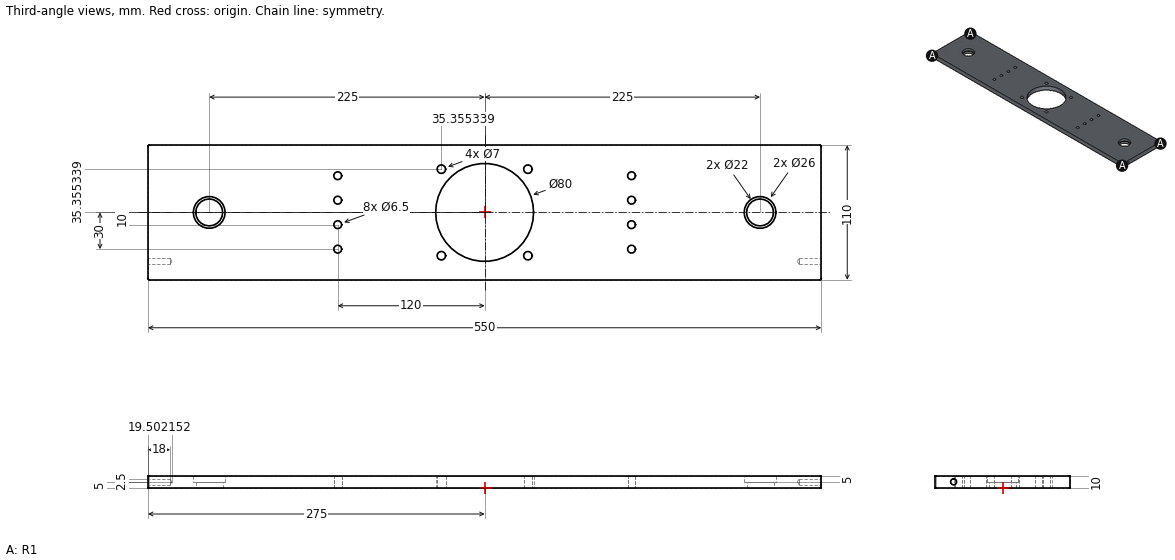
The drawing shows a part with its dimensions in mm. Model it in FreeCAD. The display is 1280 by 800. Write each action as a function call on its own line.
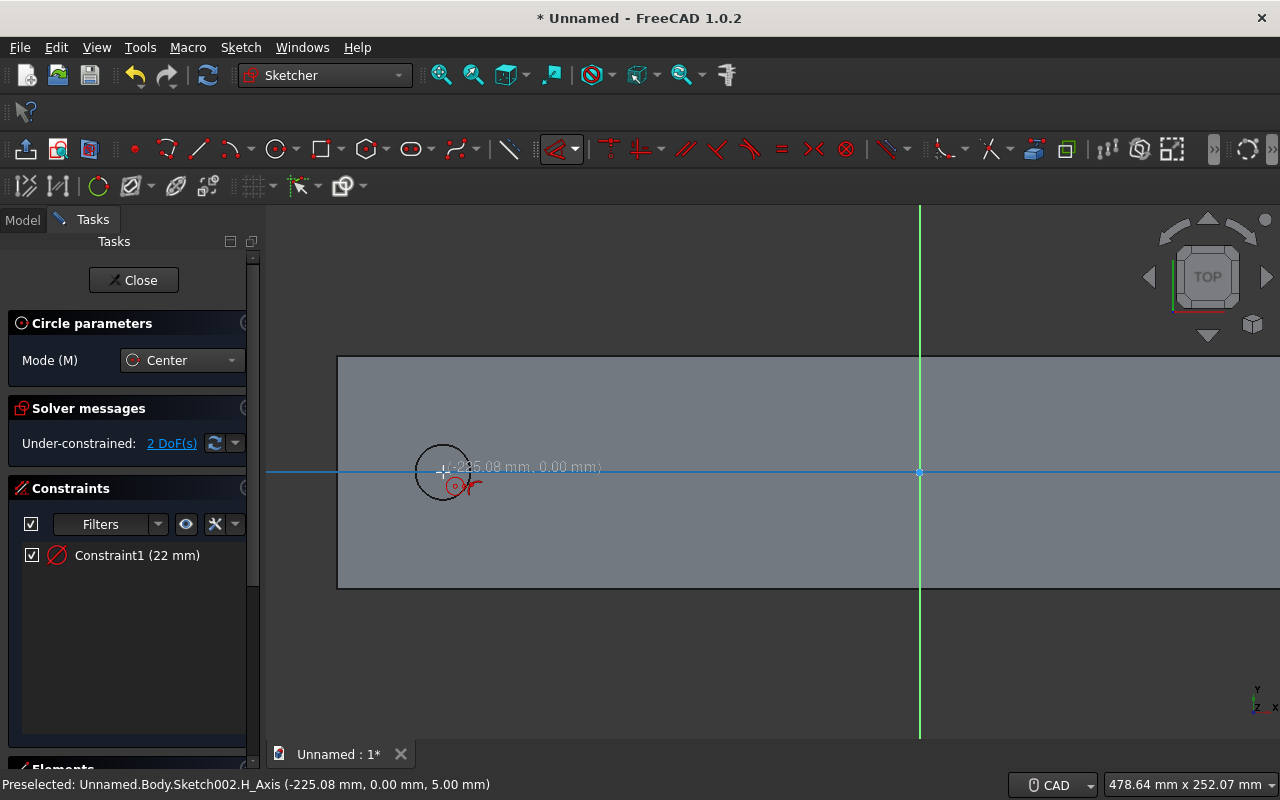
click(443, 472)
move(459, 456)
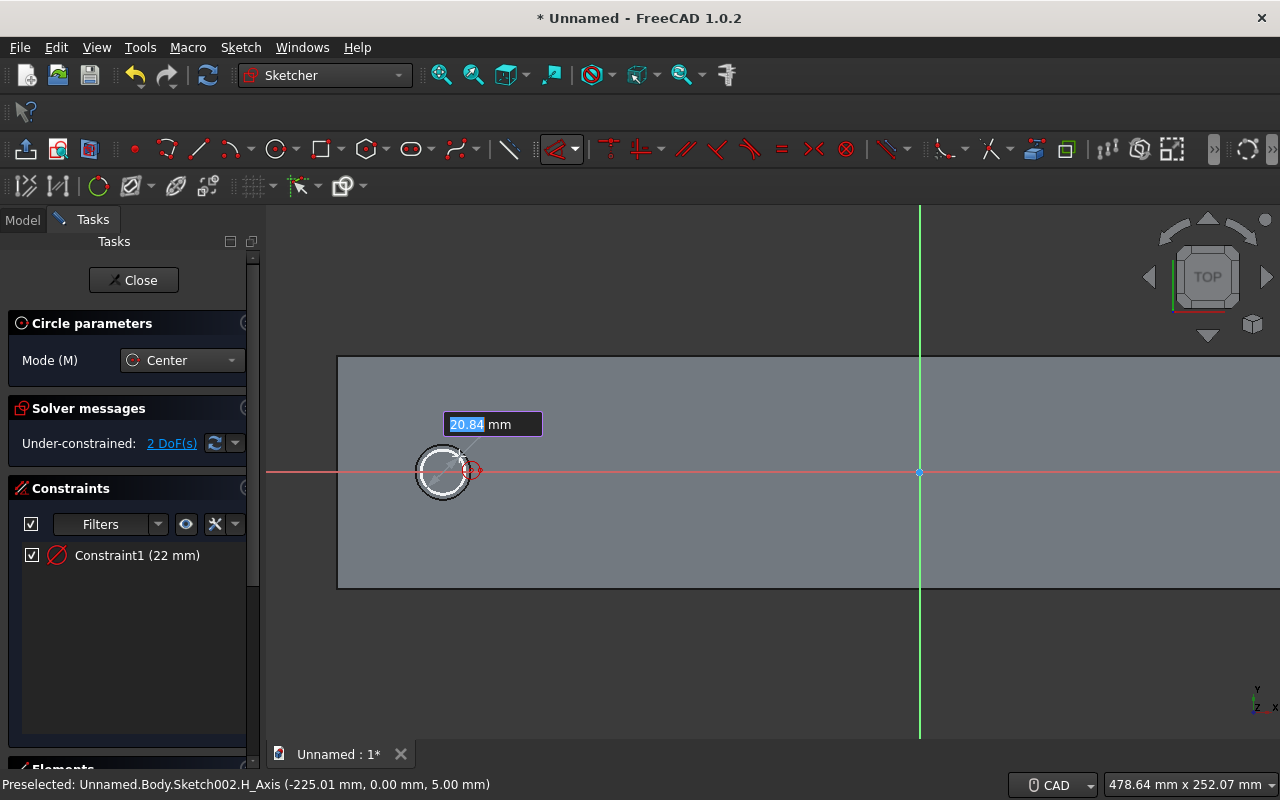
text(22)
key(Return)
key(Escape)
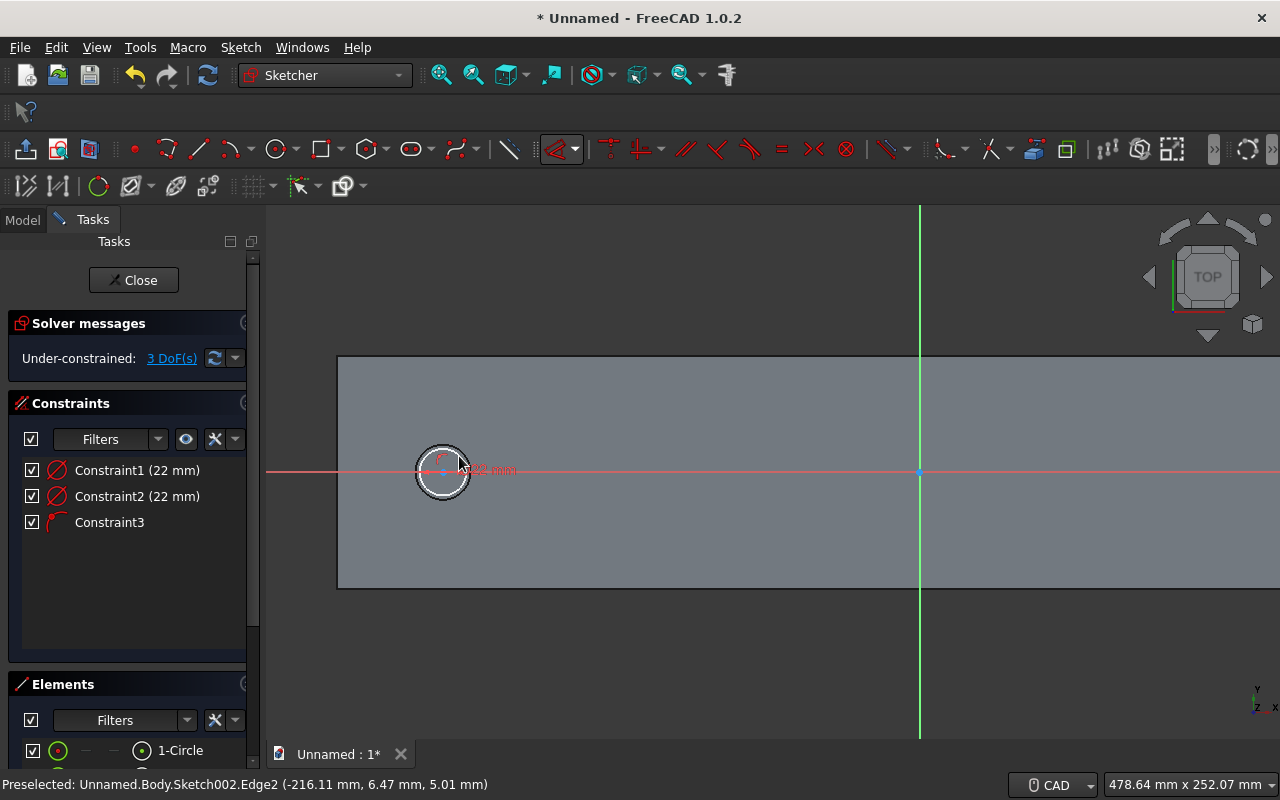
scroll(443, 472, down, 3)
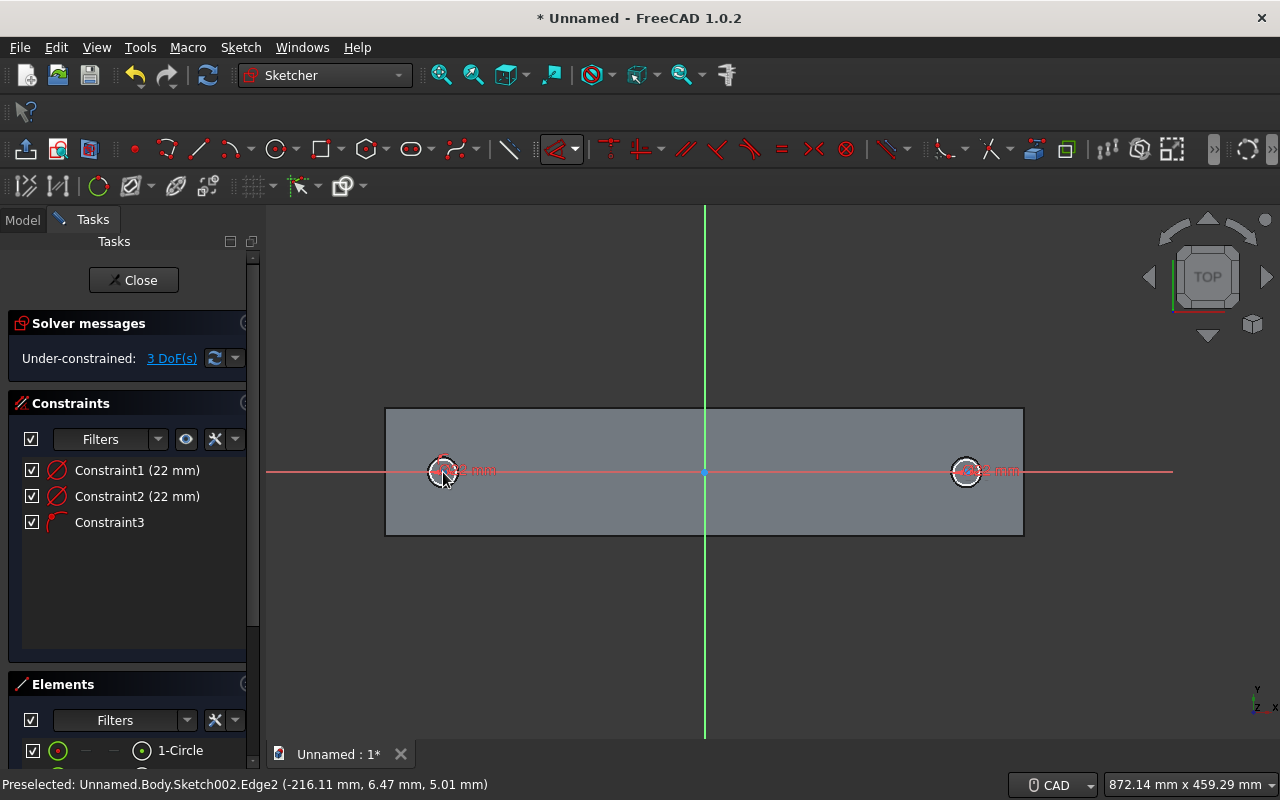
click(967, 473)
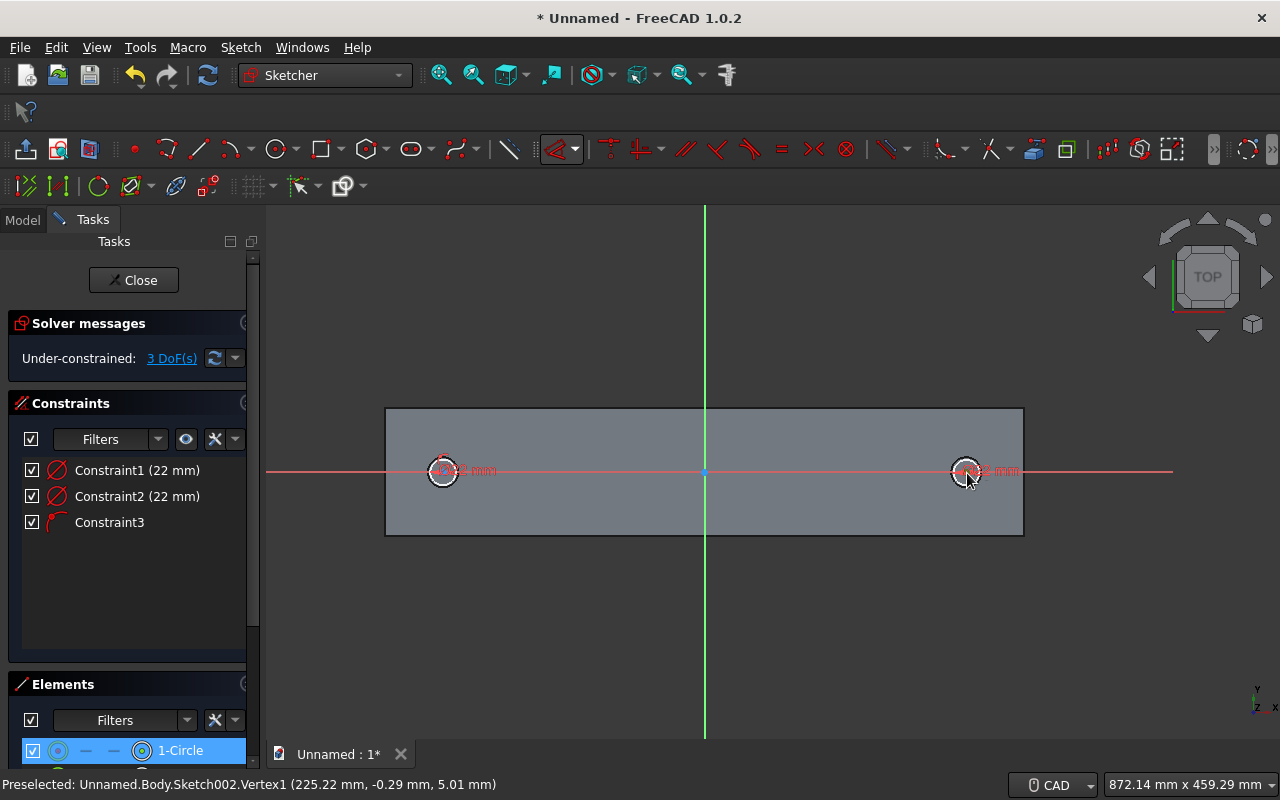
click(353, 472)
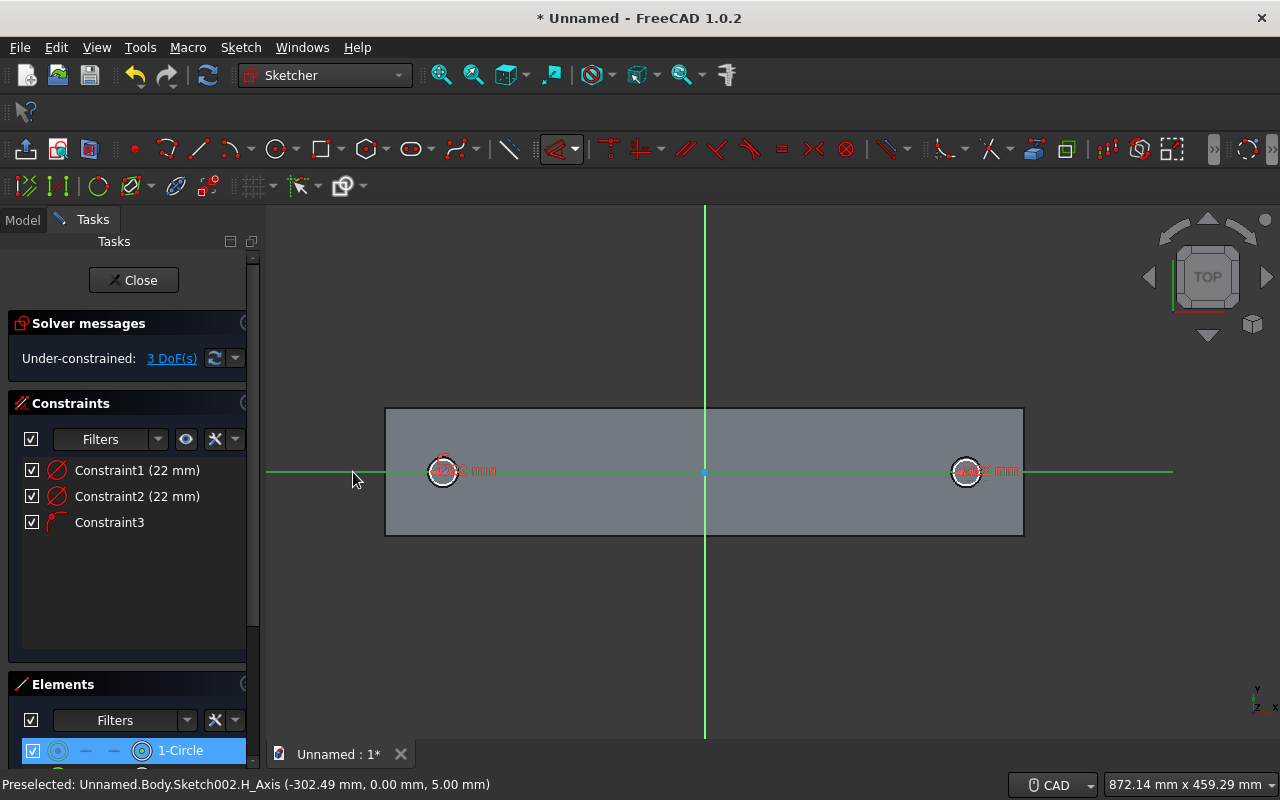
key(c)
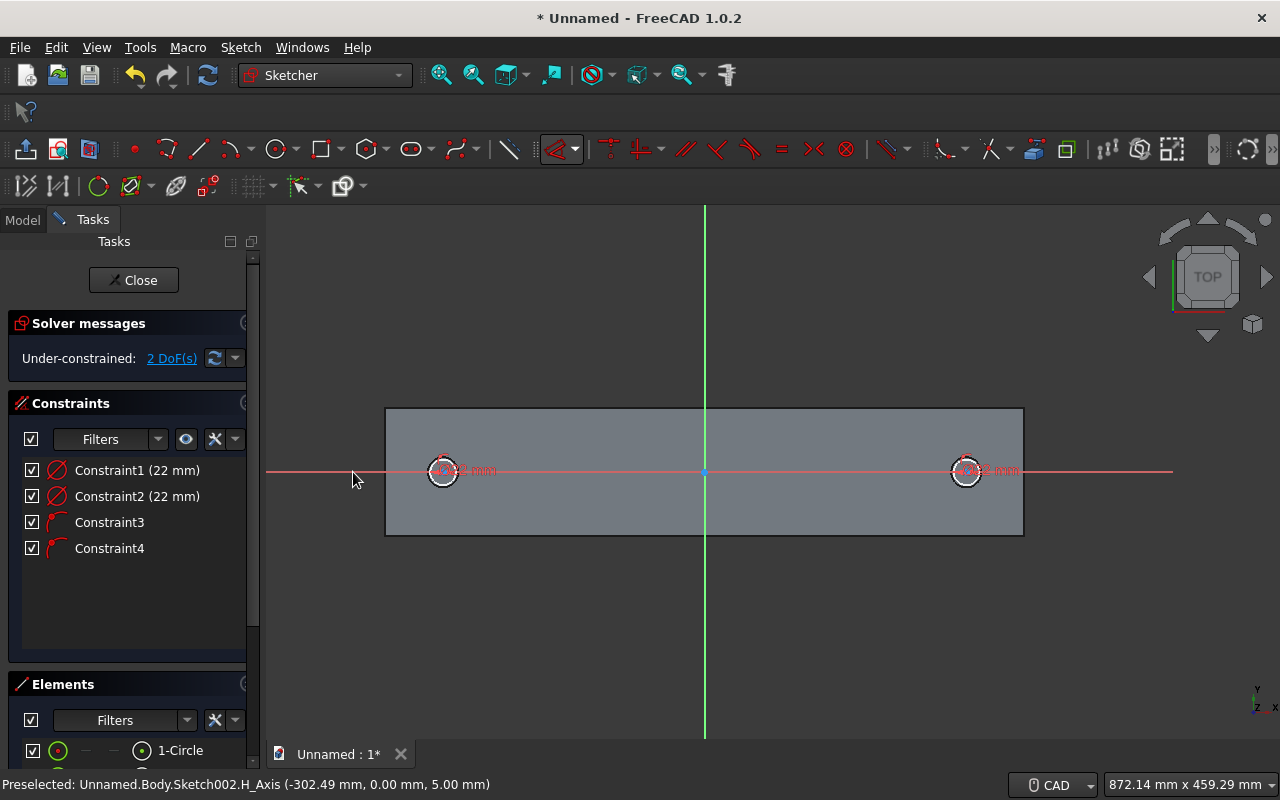
click(967, 472)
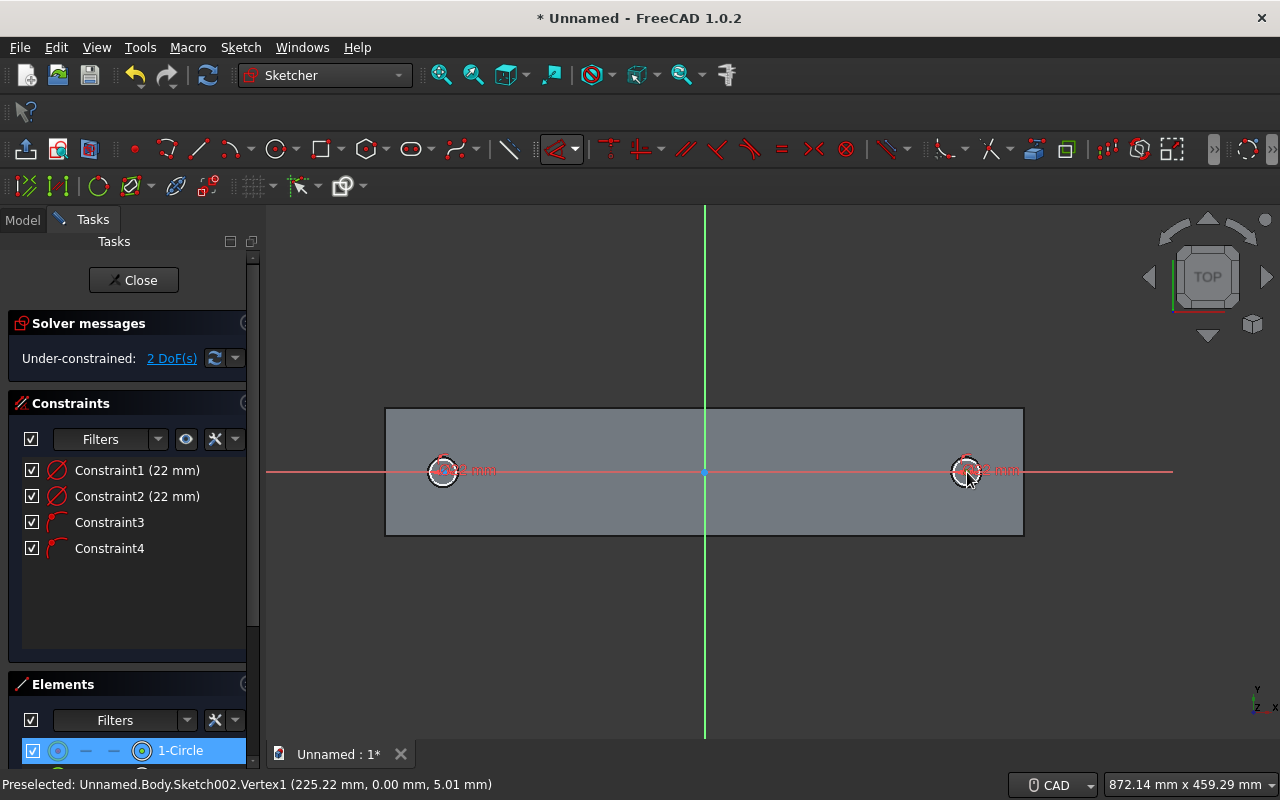
key(l)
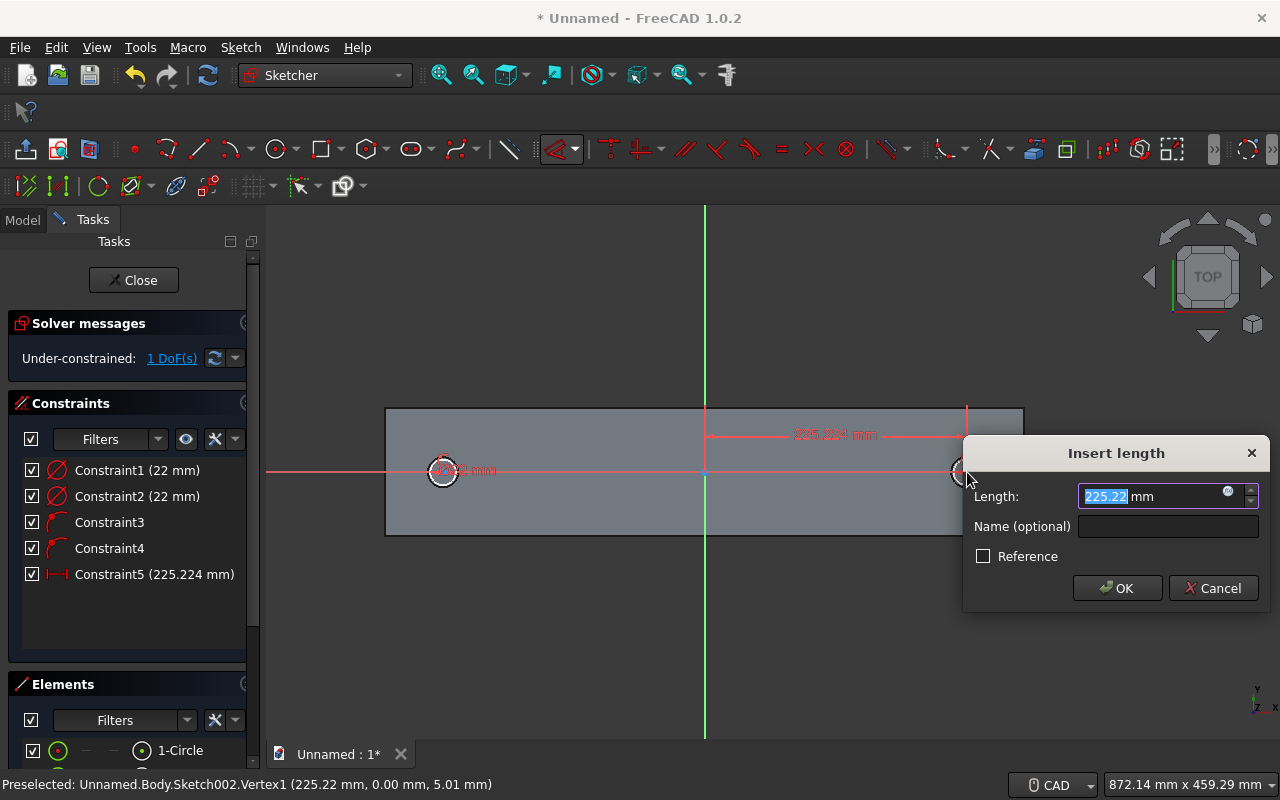
text(225)
key(Return)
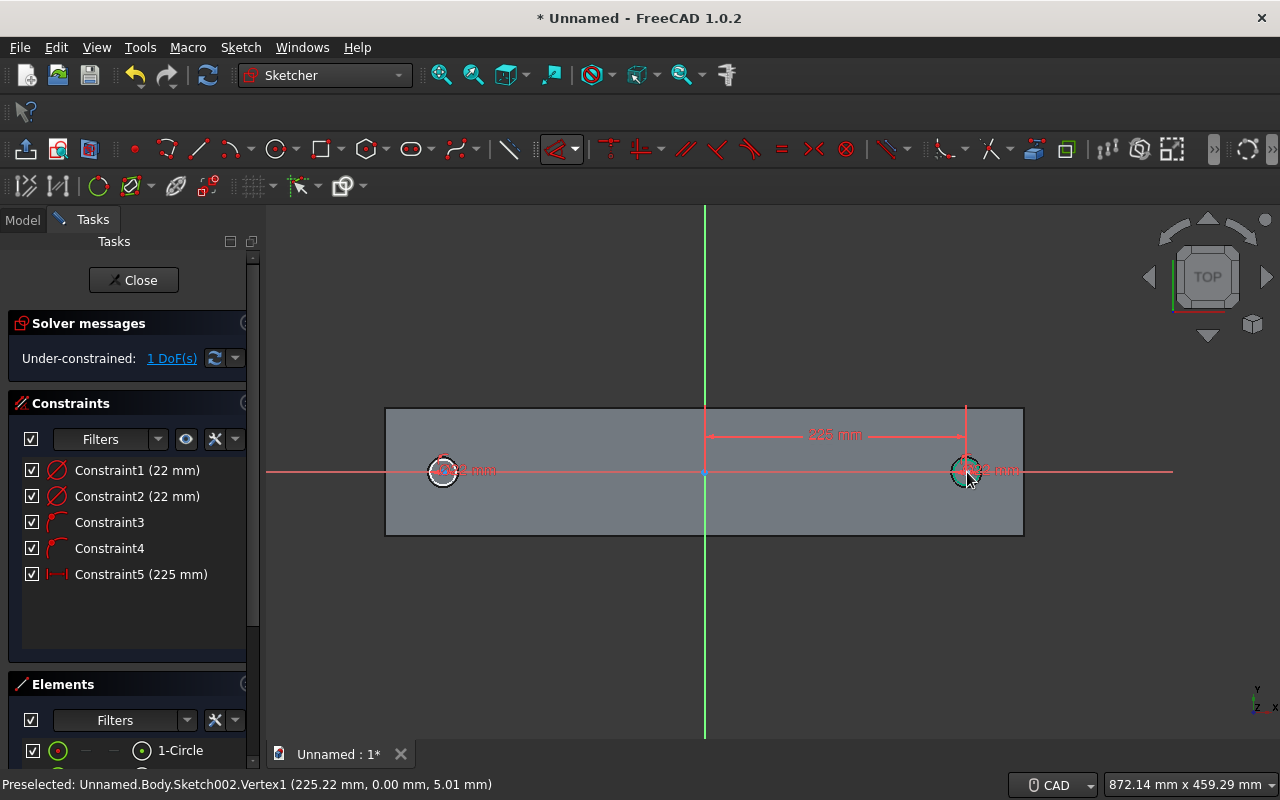
click(443, 472)